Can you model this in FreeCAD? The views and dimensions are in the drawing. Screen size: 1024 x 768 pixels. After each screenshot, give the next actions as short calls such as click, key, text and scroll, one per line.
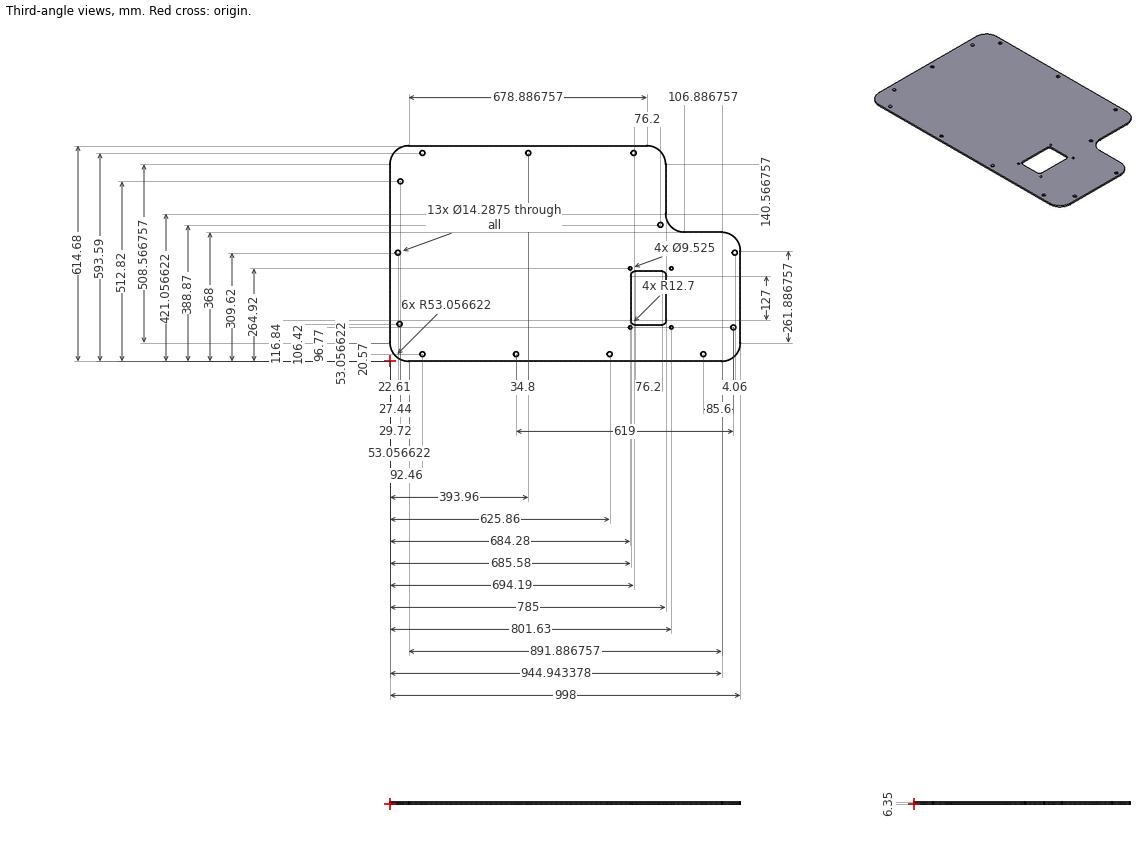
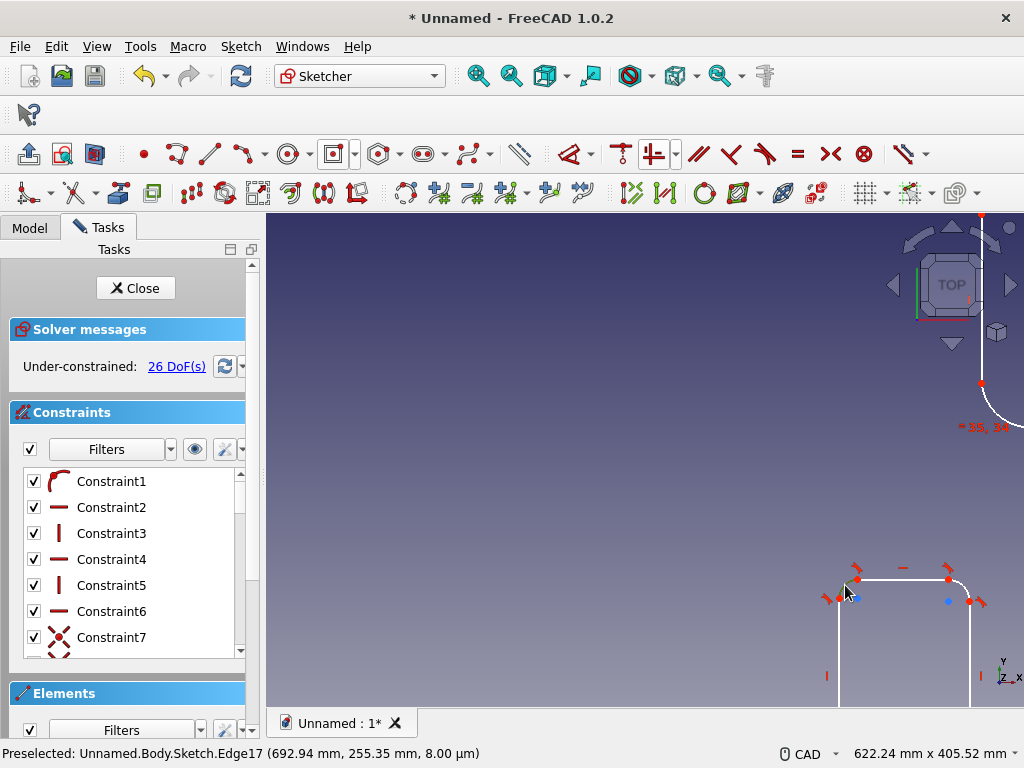
scroll(561, 434, down, 6)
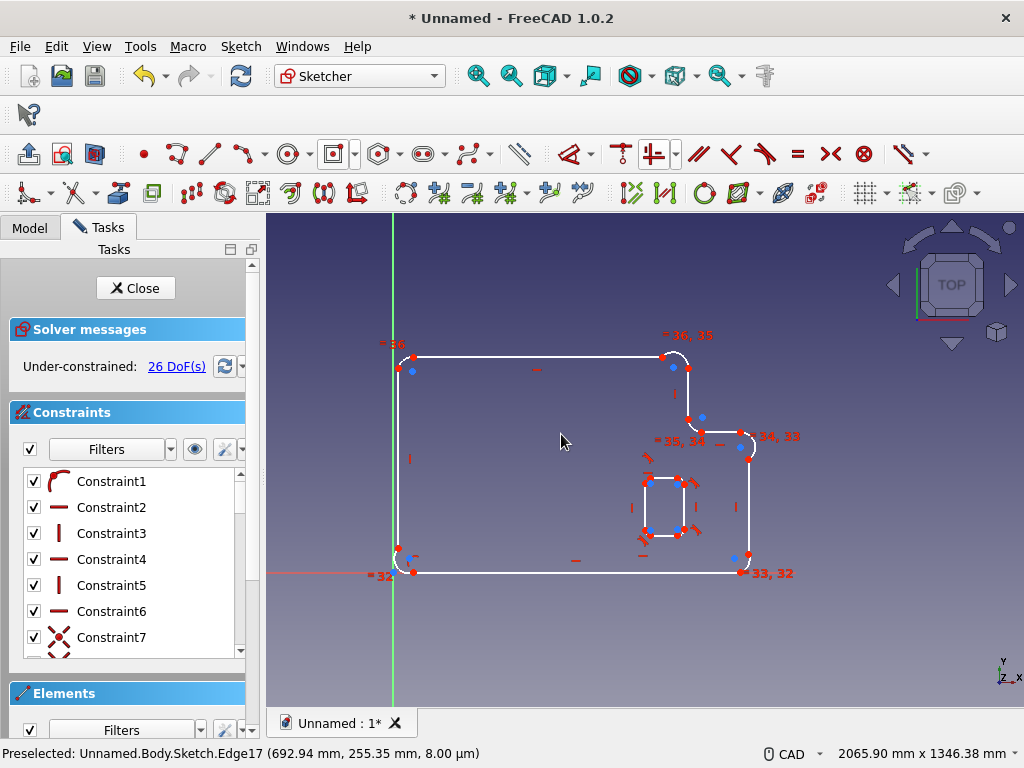
scroll(684, 482, up, 8)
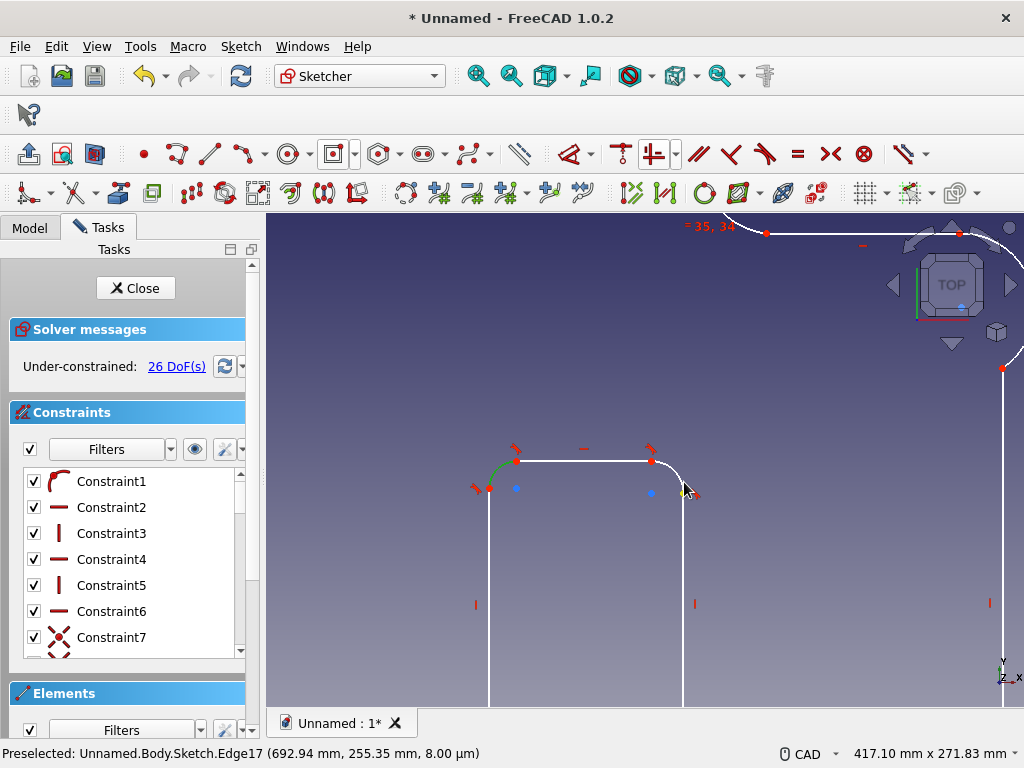
click(680, 479)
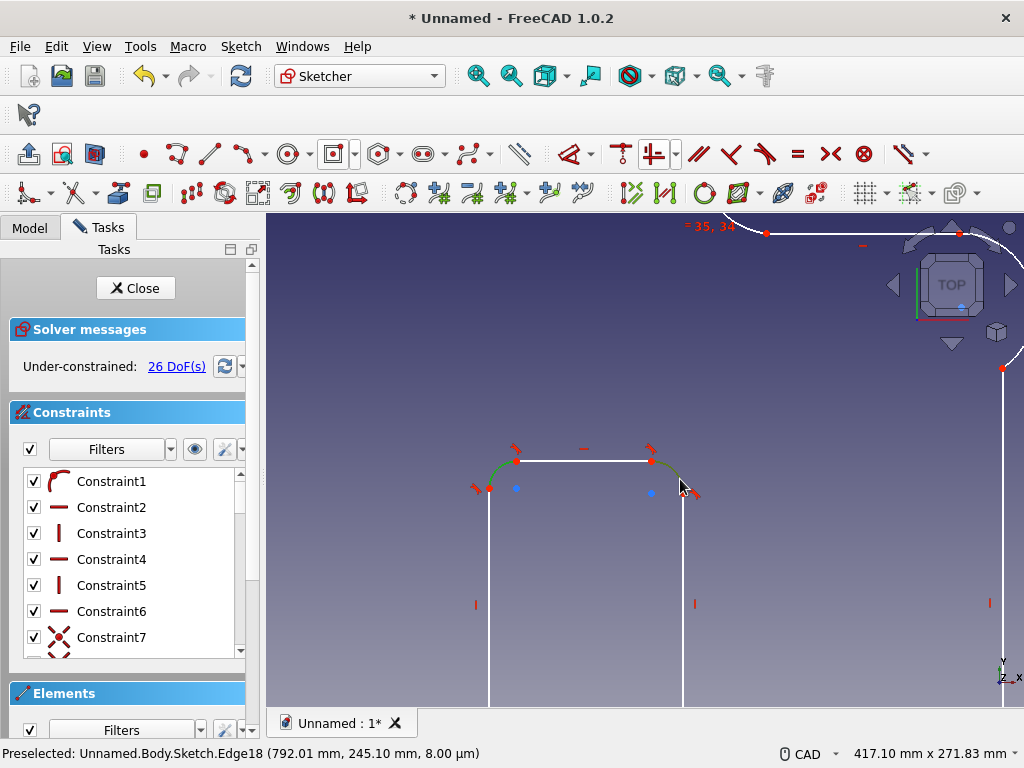
scroll(684, 482, down, 8)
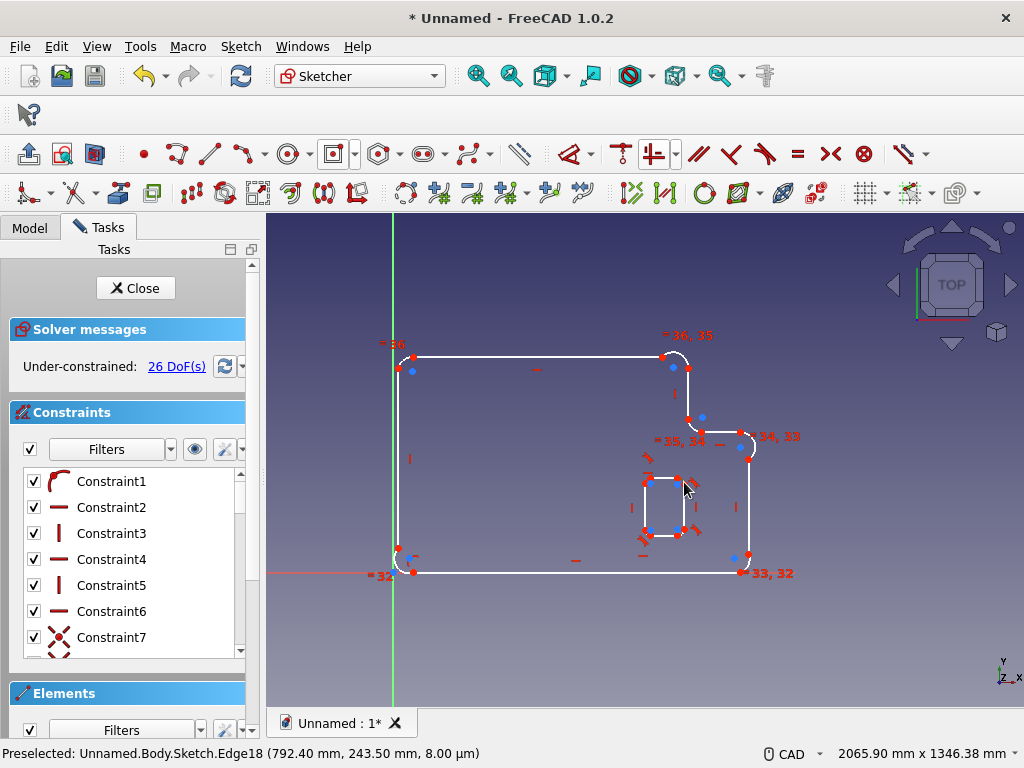
scroll(681, 535, up, 8)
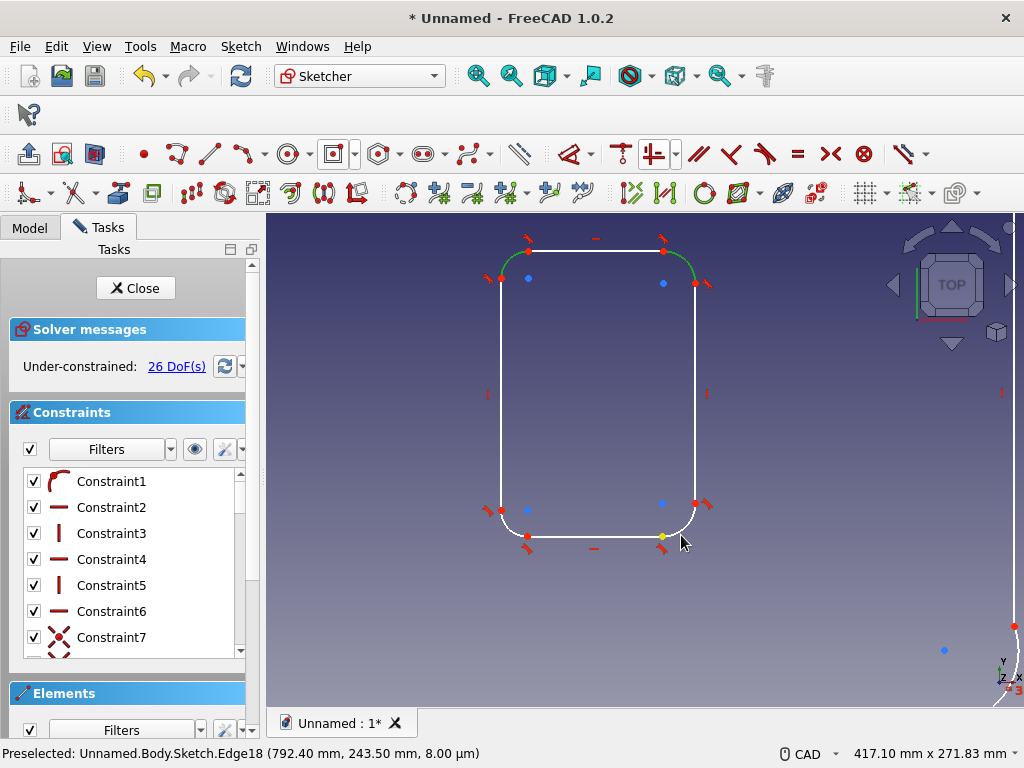
click(677, 533)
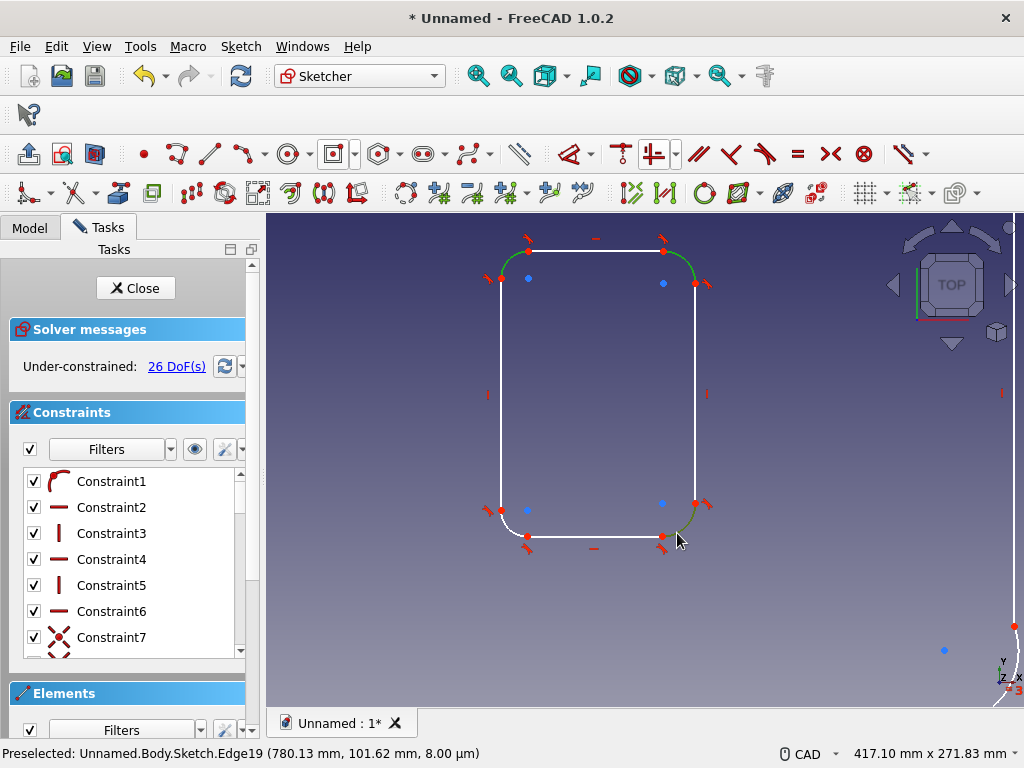
click(504, 522)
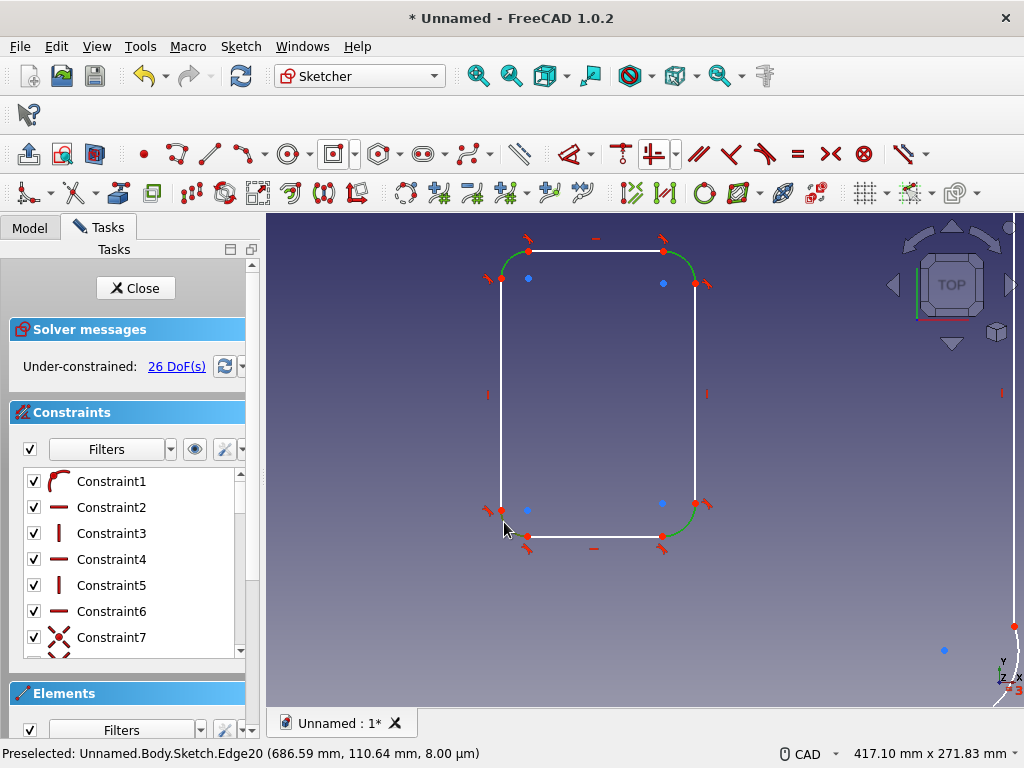
click(798, 154)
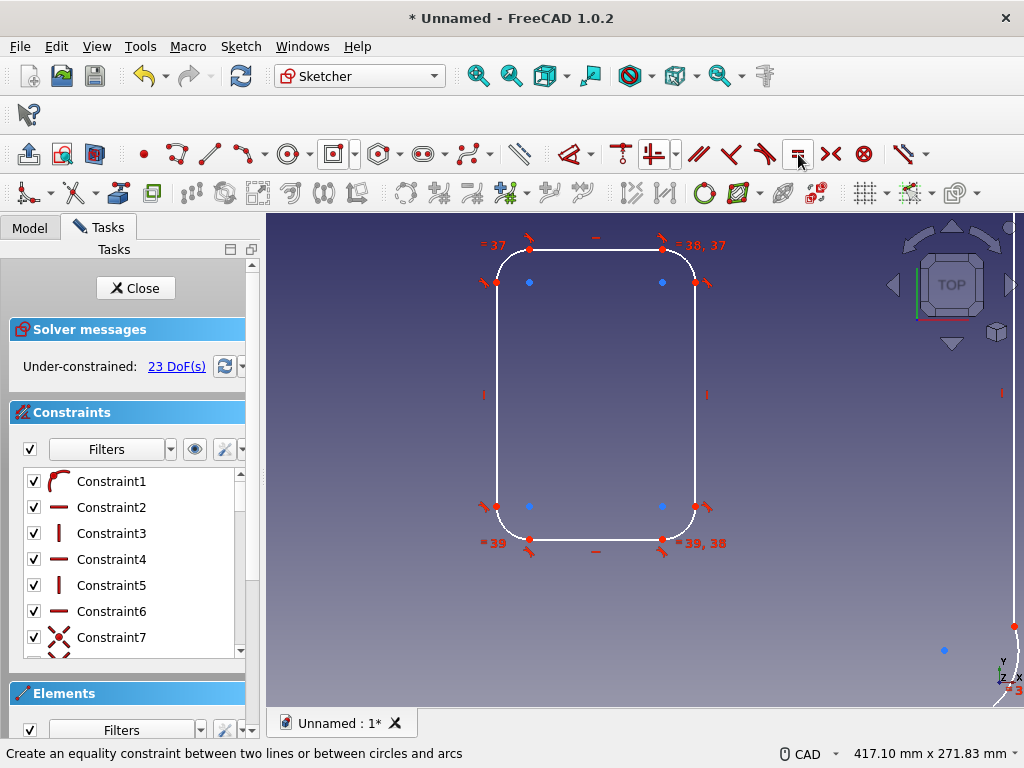
scroll(681, 536, down, 8)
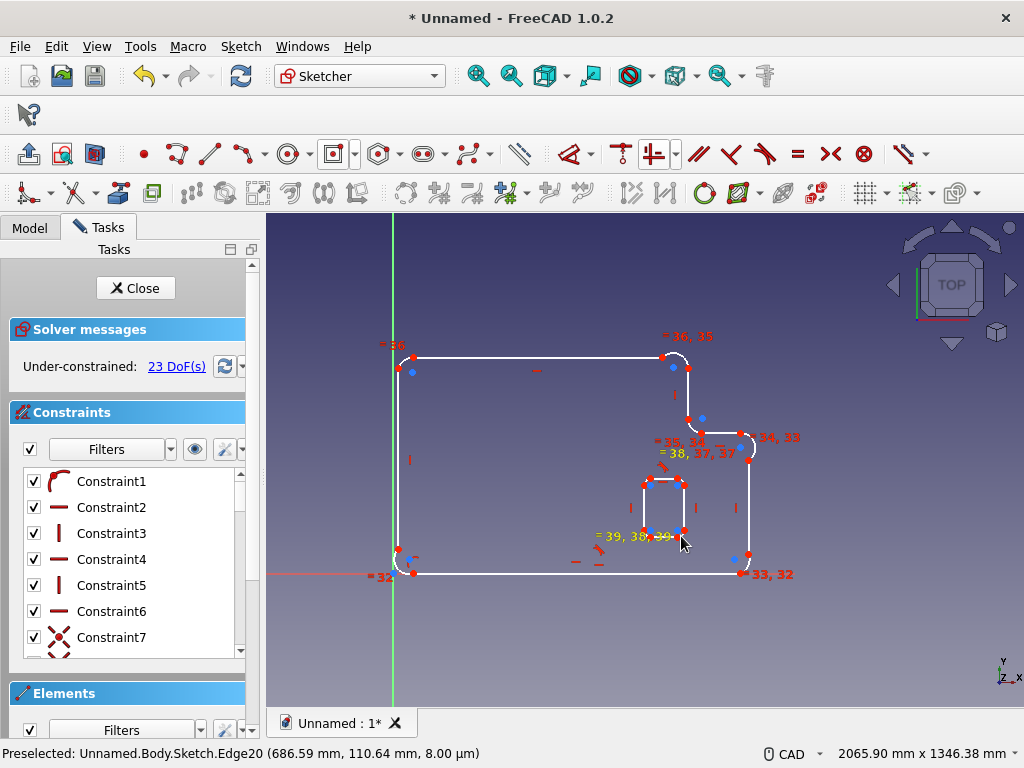
scroll(396, 567, up, 8)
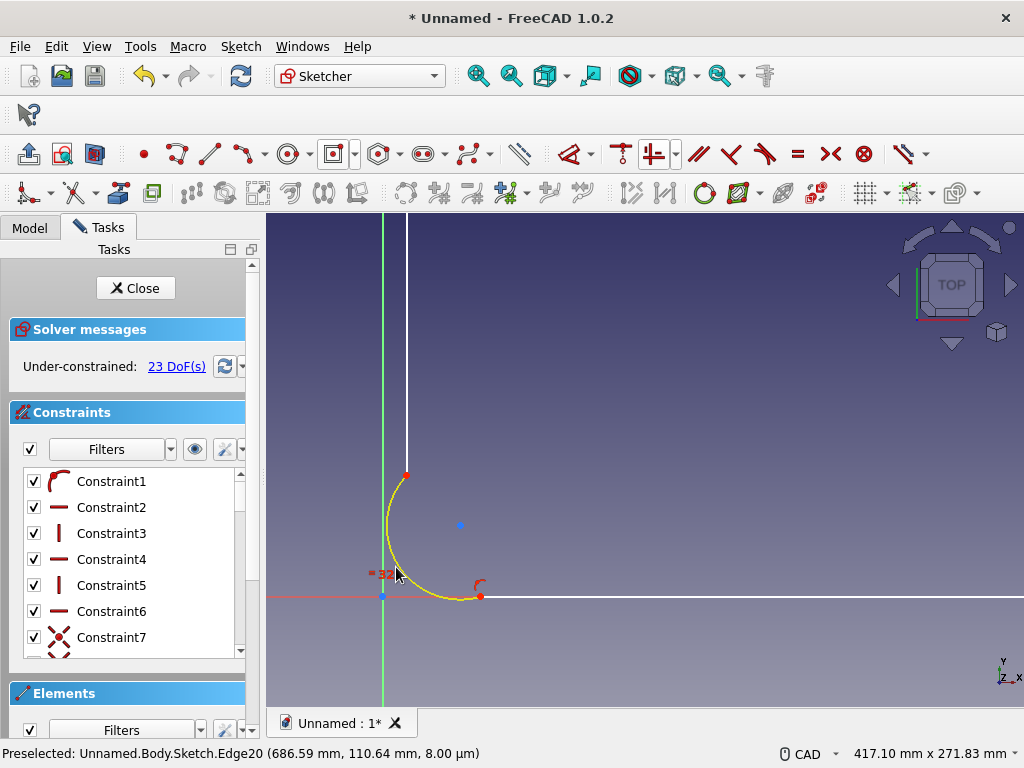
click(398, 564)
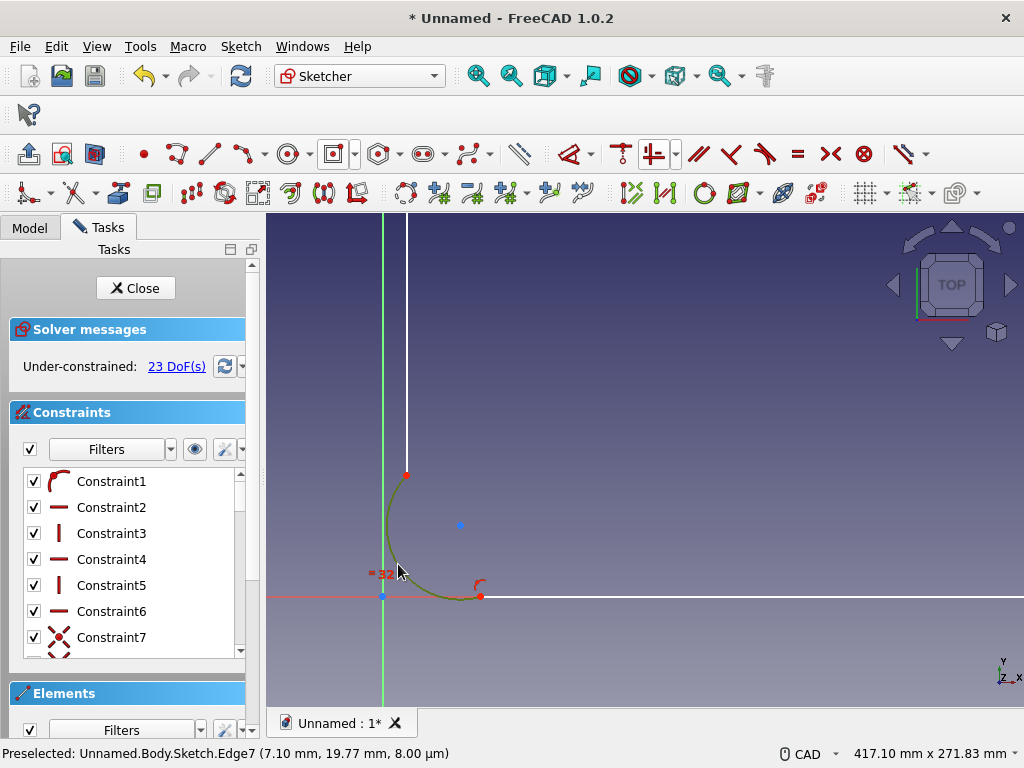
key(k)
key(r)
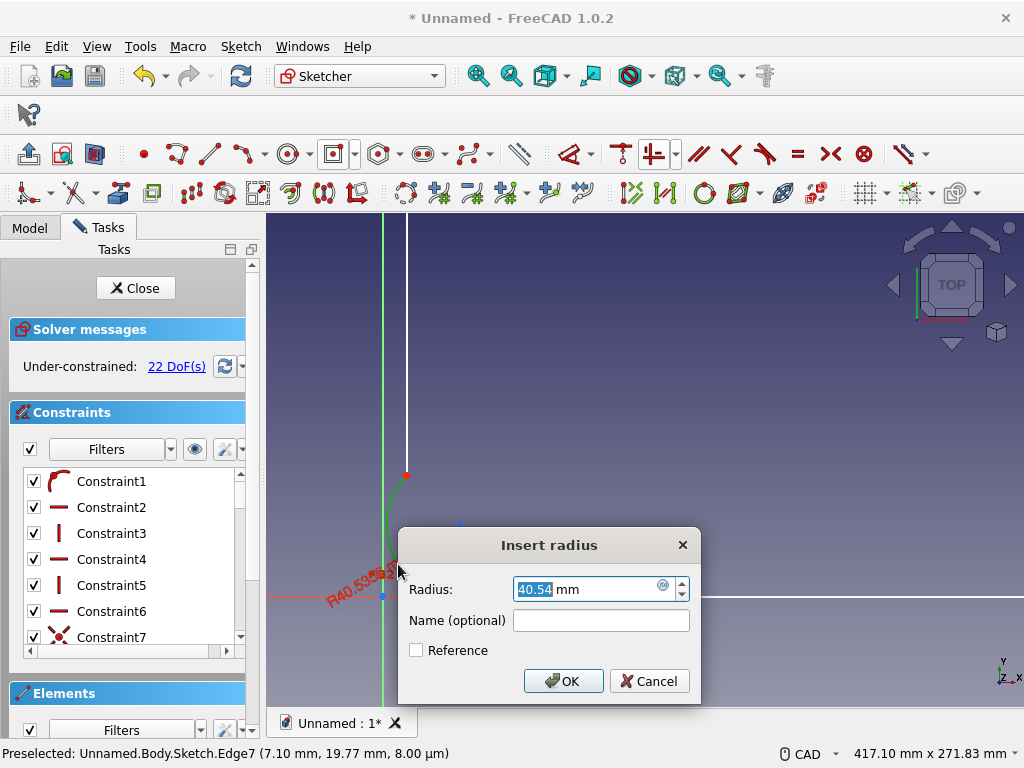
text(53.056622)
key(Return)